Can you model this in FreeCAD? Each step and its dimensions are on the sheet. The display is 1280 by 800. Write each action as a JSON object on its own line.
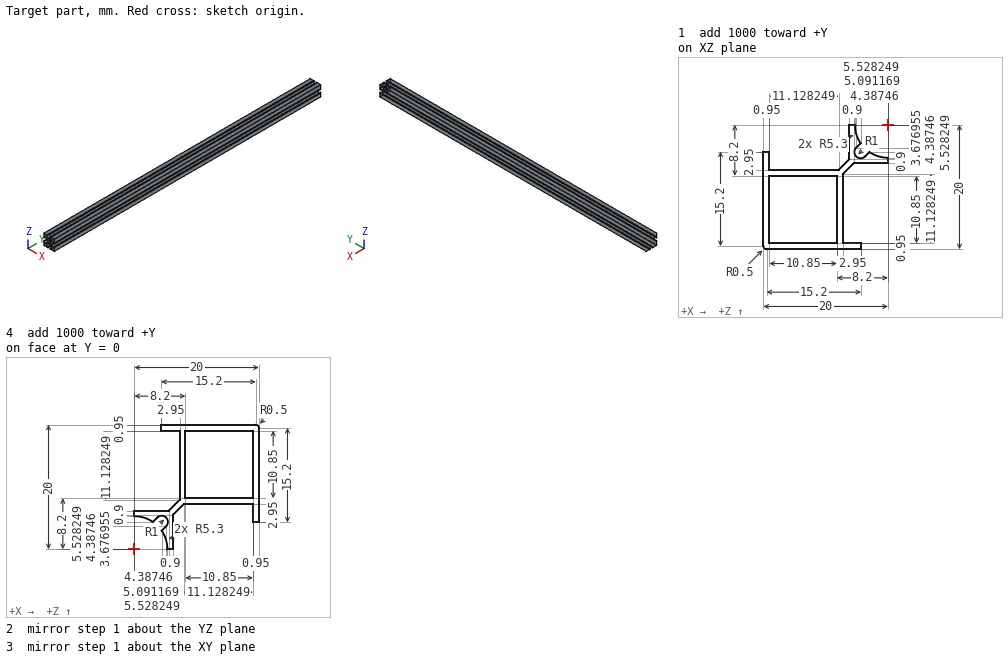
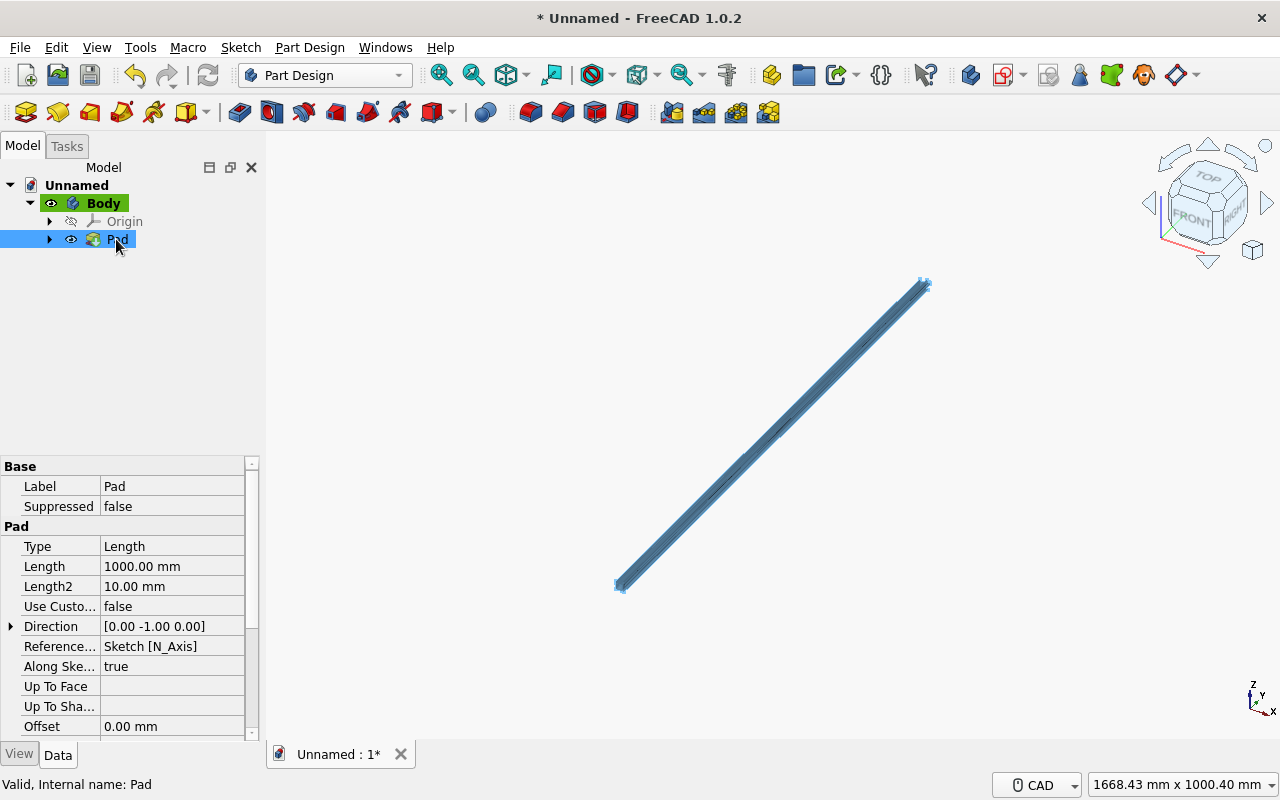
{"action": "left_click", "coordinate": [672, 112]}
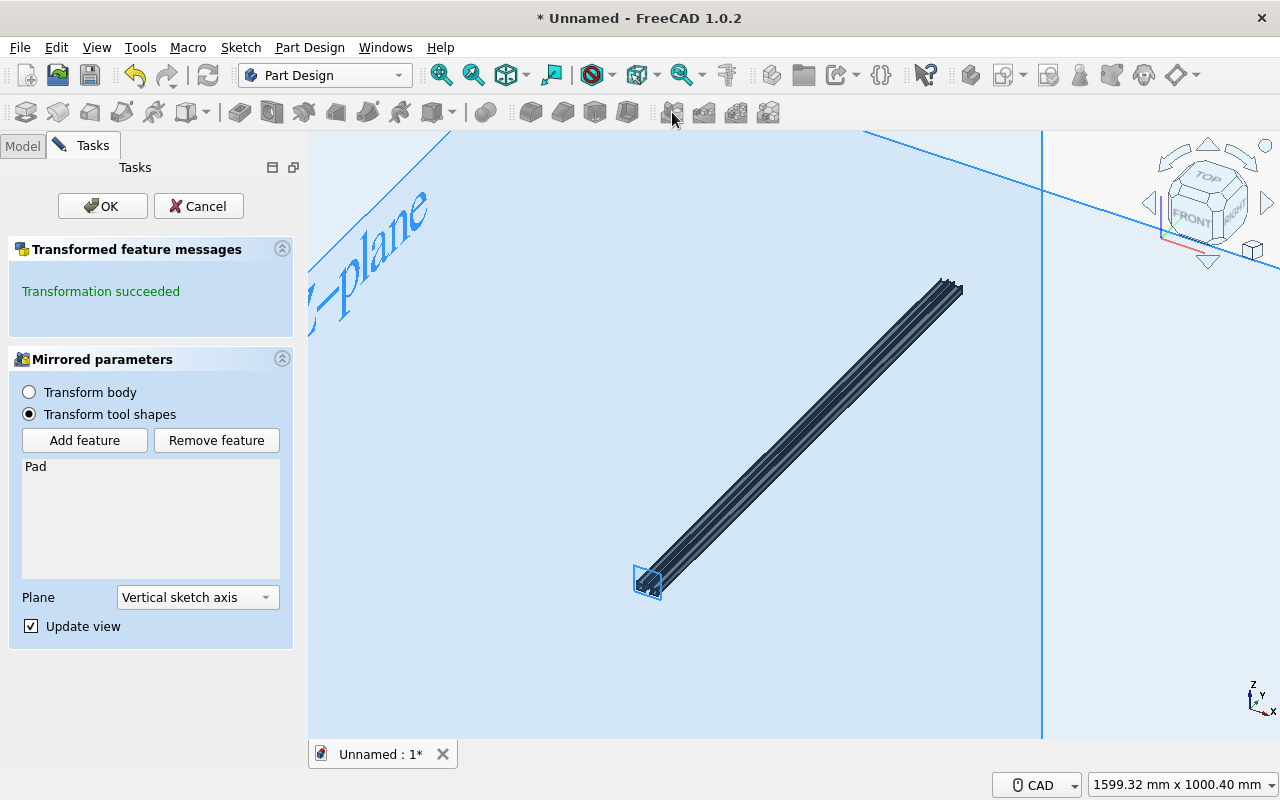
{"action": "left_click", "coordinate": [198, 598]}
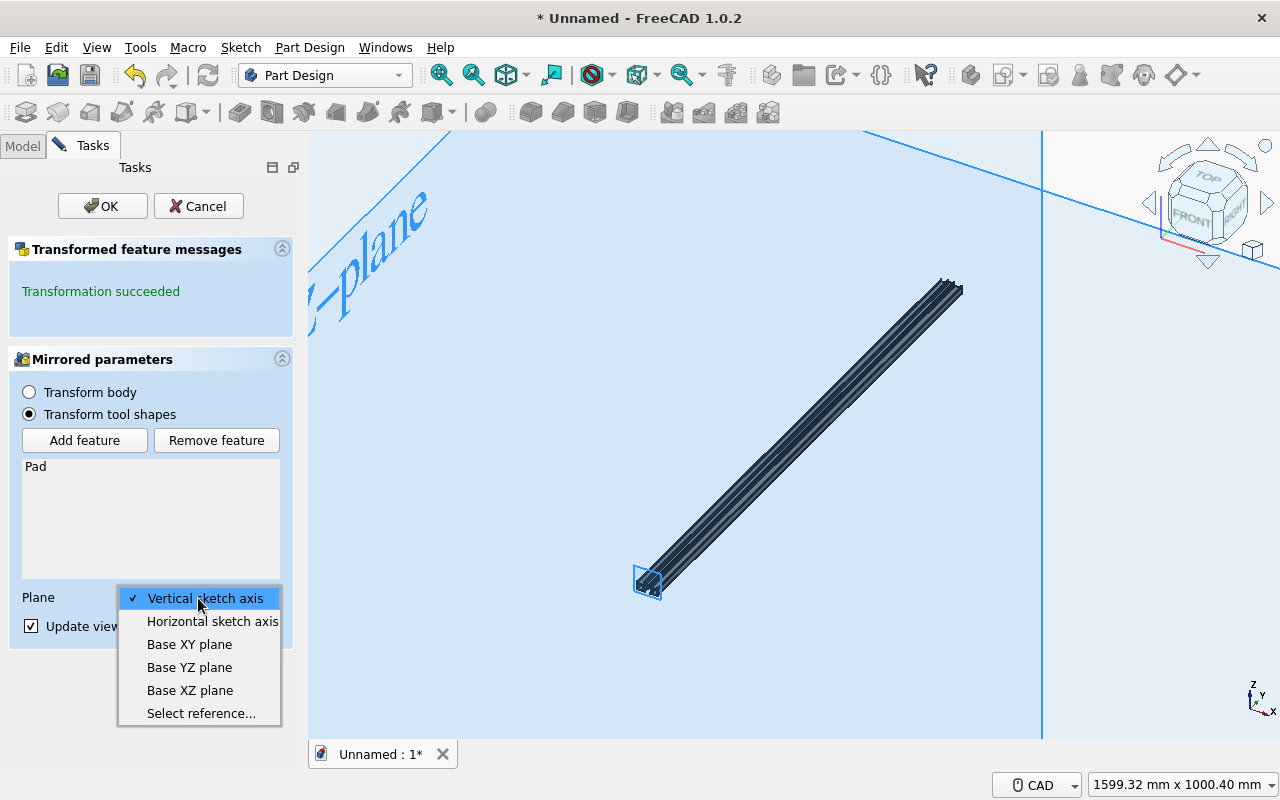
{"action": "left_click", "coordinate": [198, 668]}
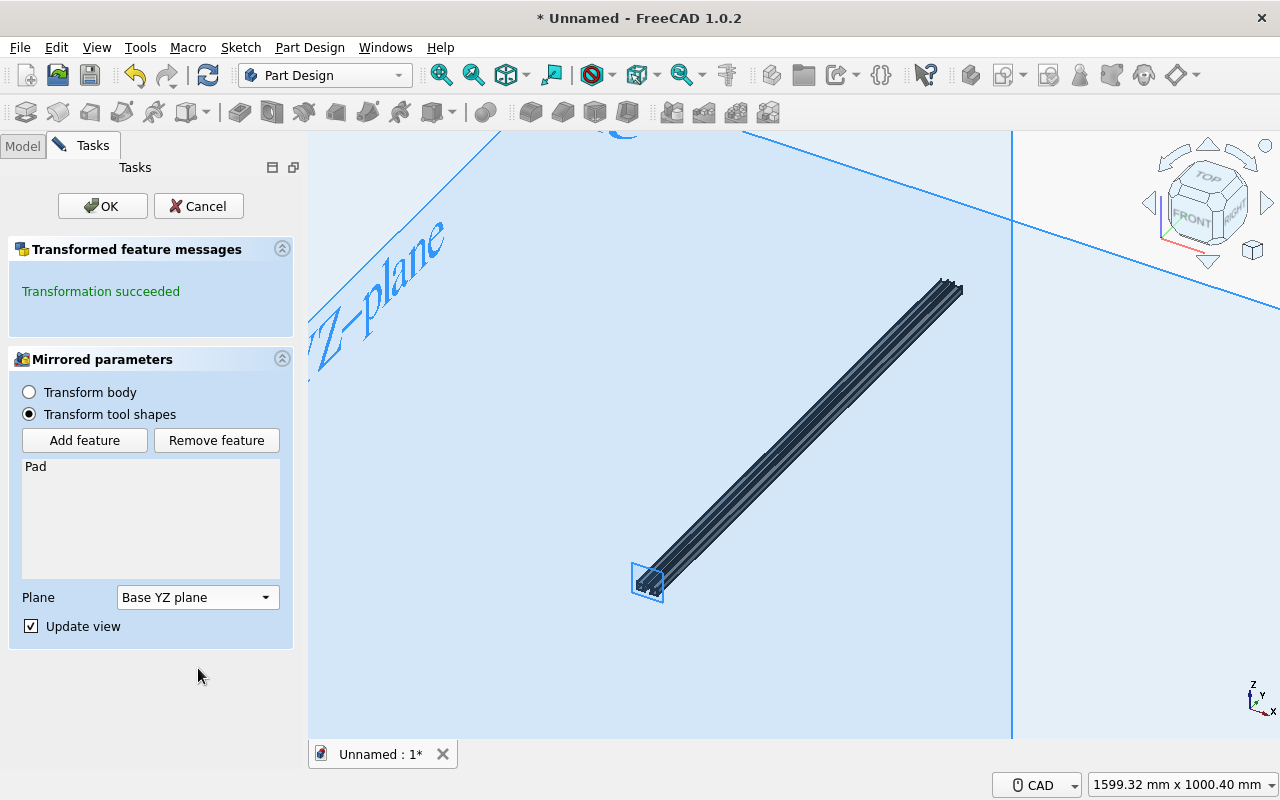
{"action": "left_click", "coordinate": [103, 206]}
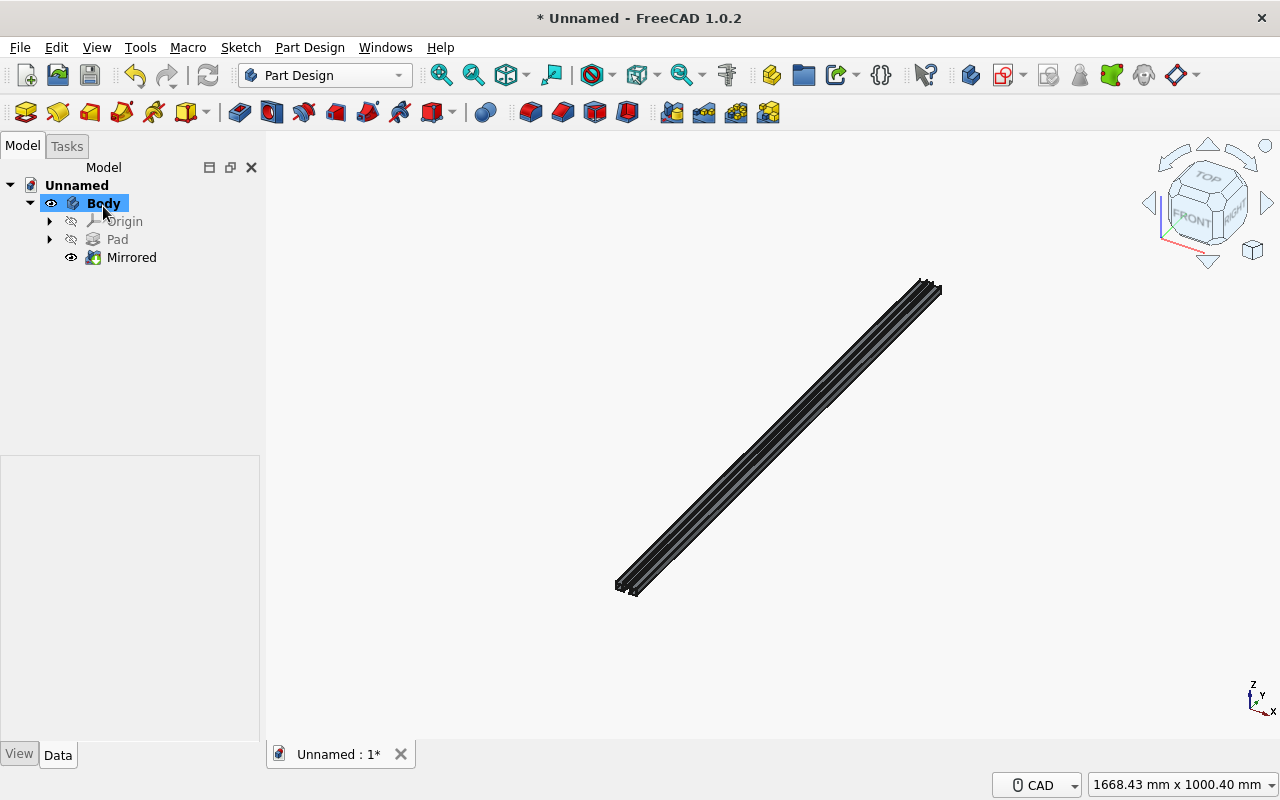
{"action": "left_click", "coordinate": [116, 239]}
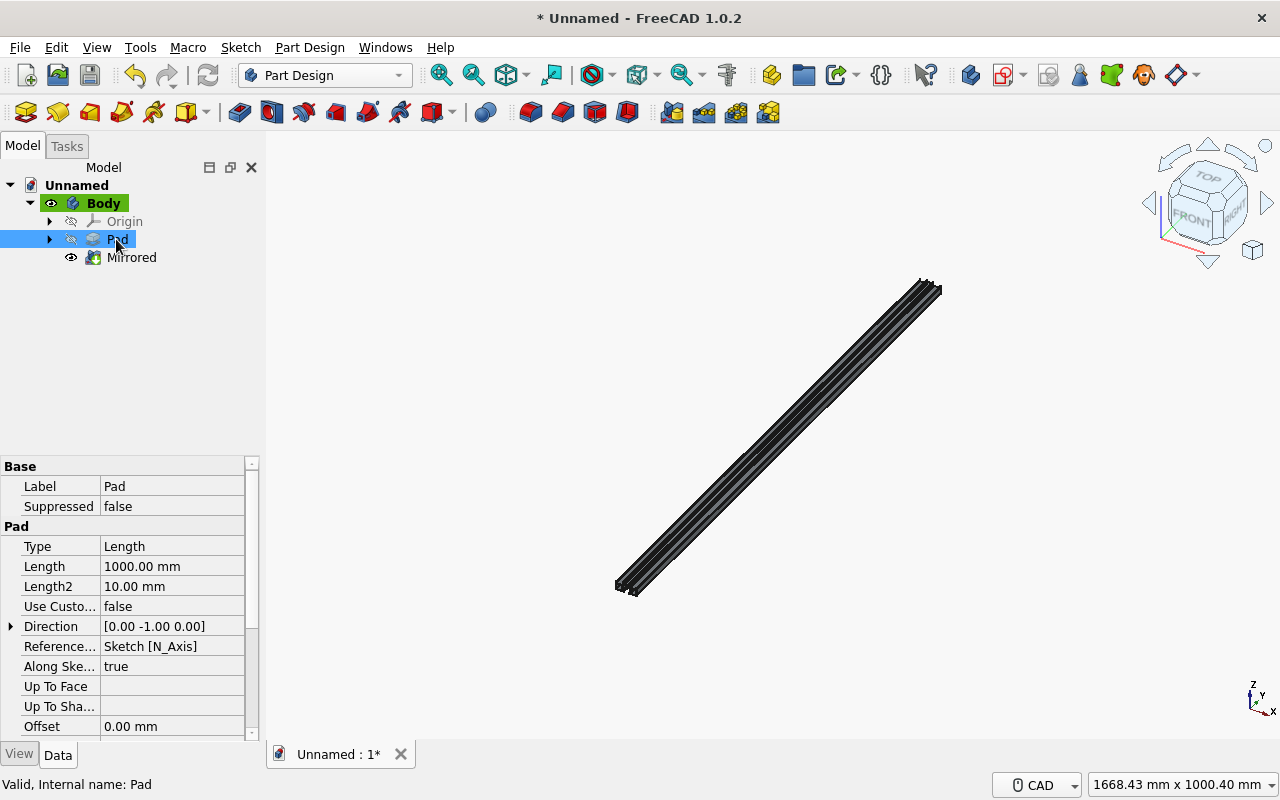
{"action": "left_click", "coordinate": [672, 112]}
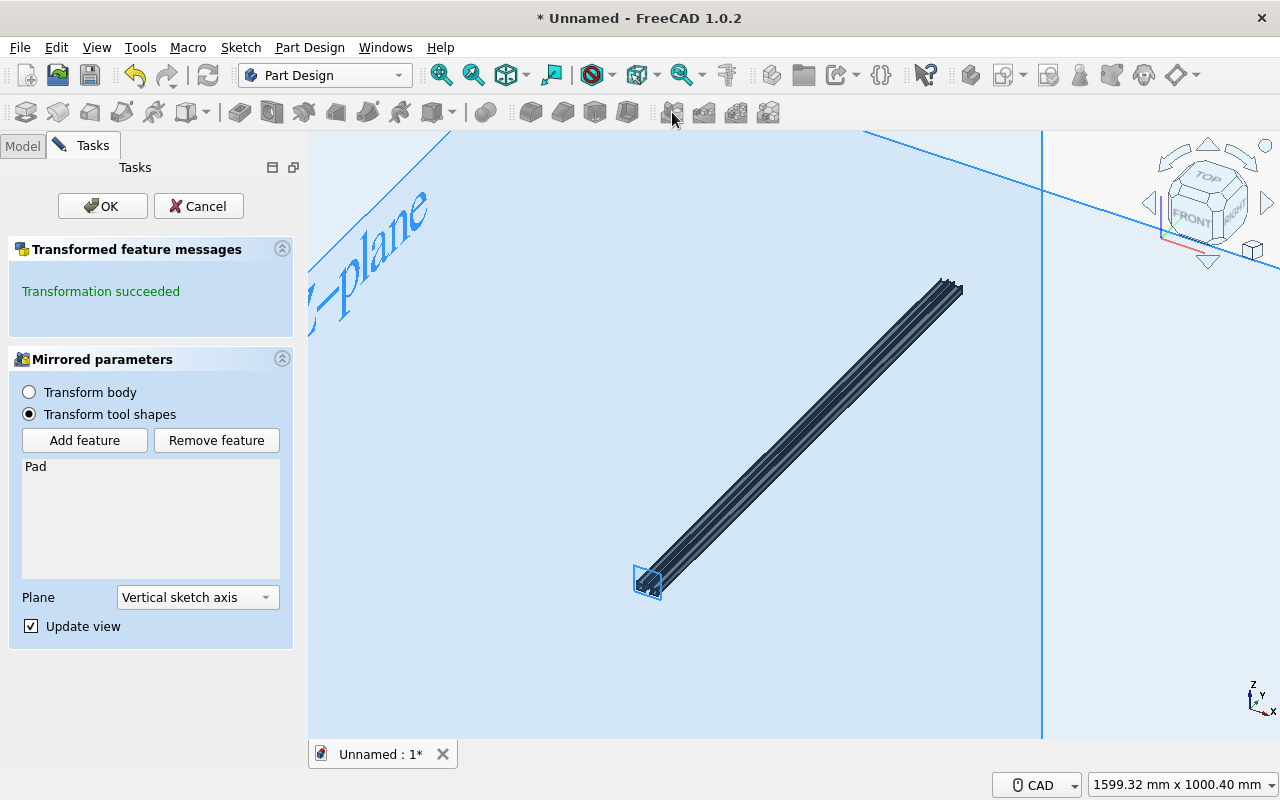
{"action": "left_click", "coordinate": [198, 598]}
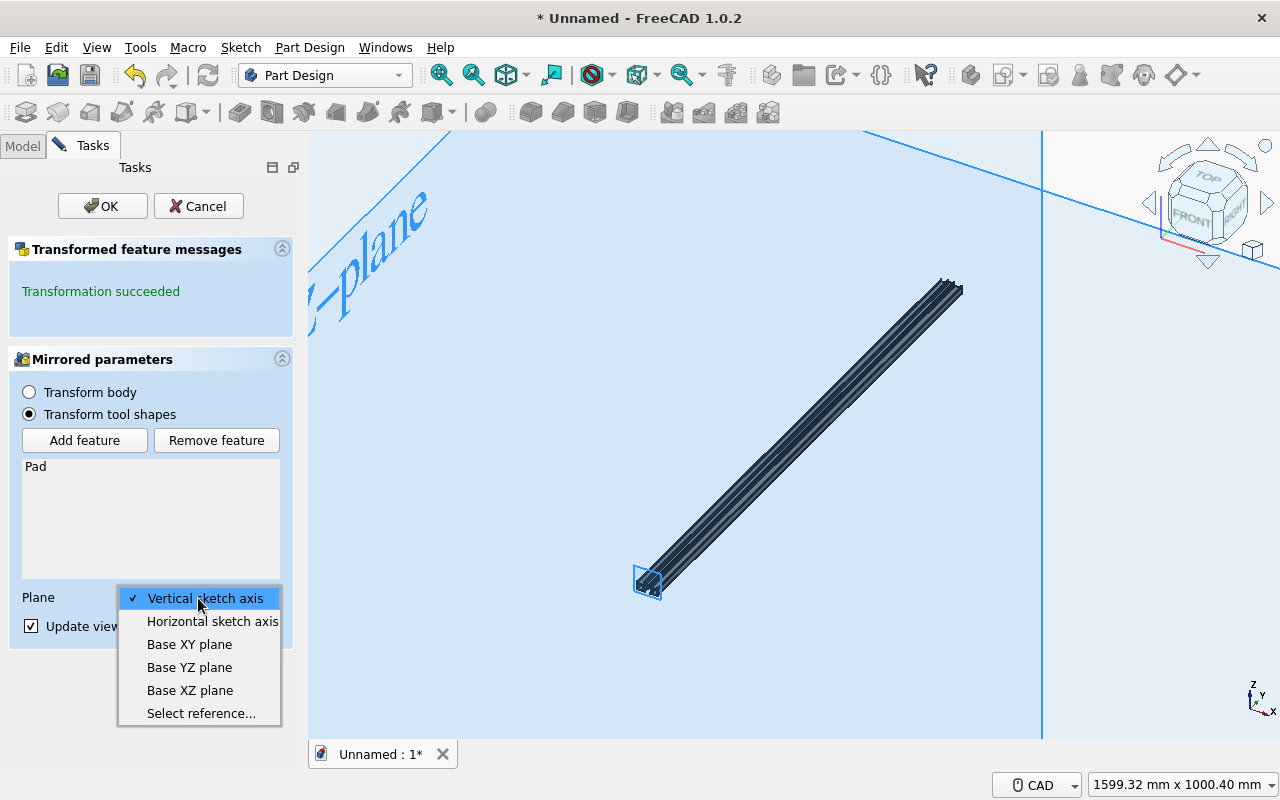
{"action": "left_click", "coordinate": [198, 644]}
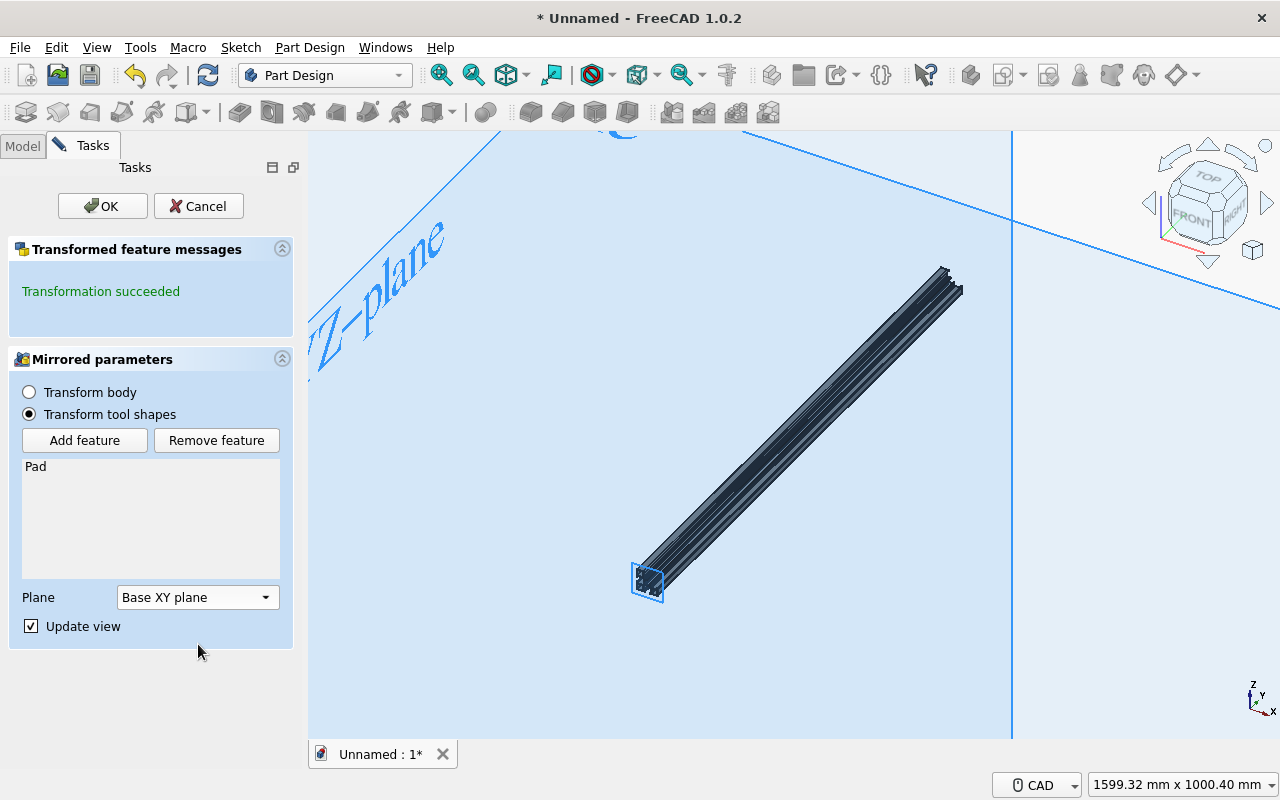
{"action": "left_click", "coordinate": [103, 206]}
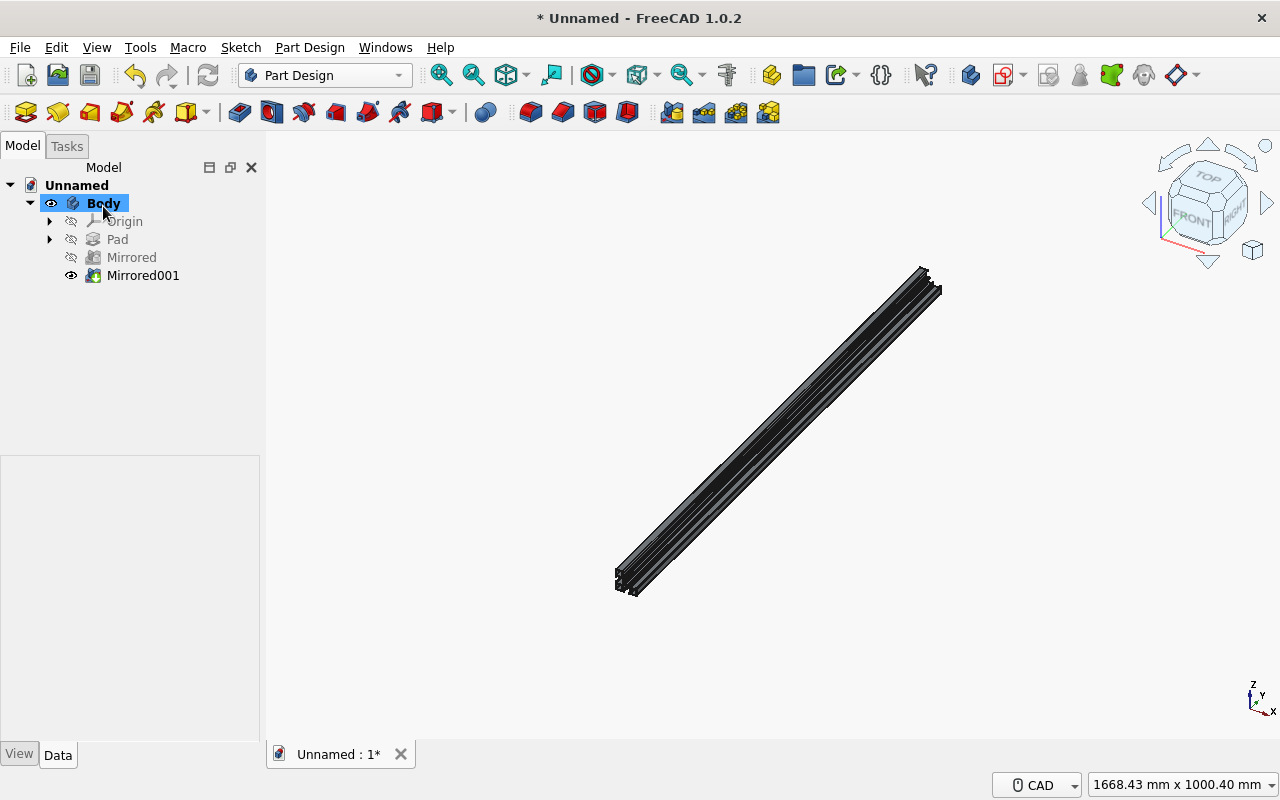
{"action": "scroll", "coordinate": [623, 578], "scroll_direction": "up", "scroll_amount": 15}